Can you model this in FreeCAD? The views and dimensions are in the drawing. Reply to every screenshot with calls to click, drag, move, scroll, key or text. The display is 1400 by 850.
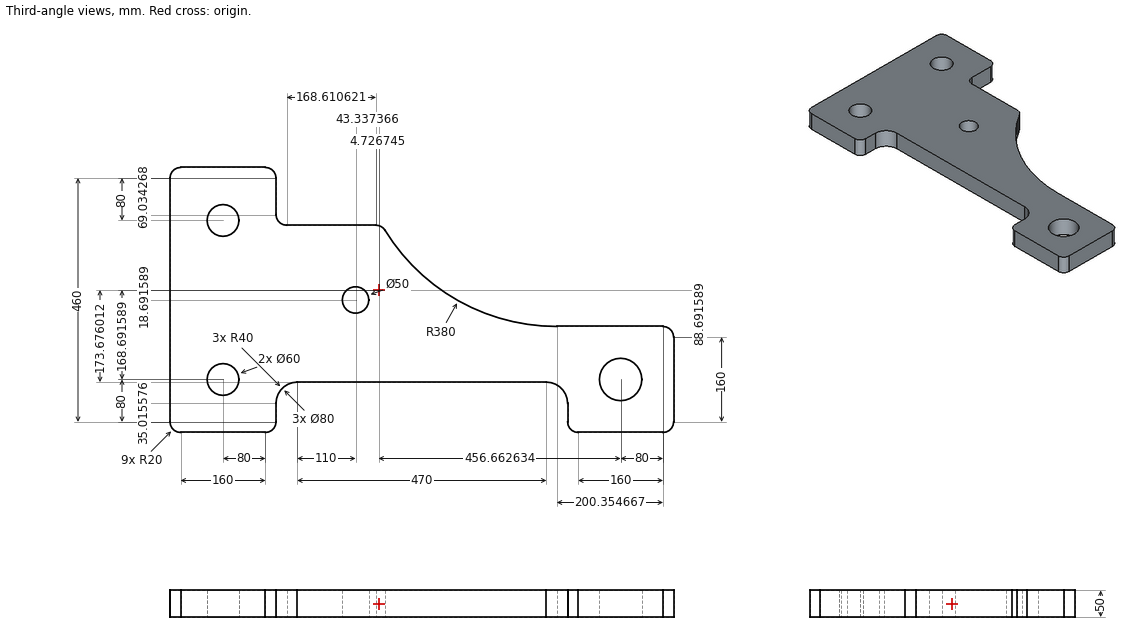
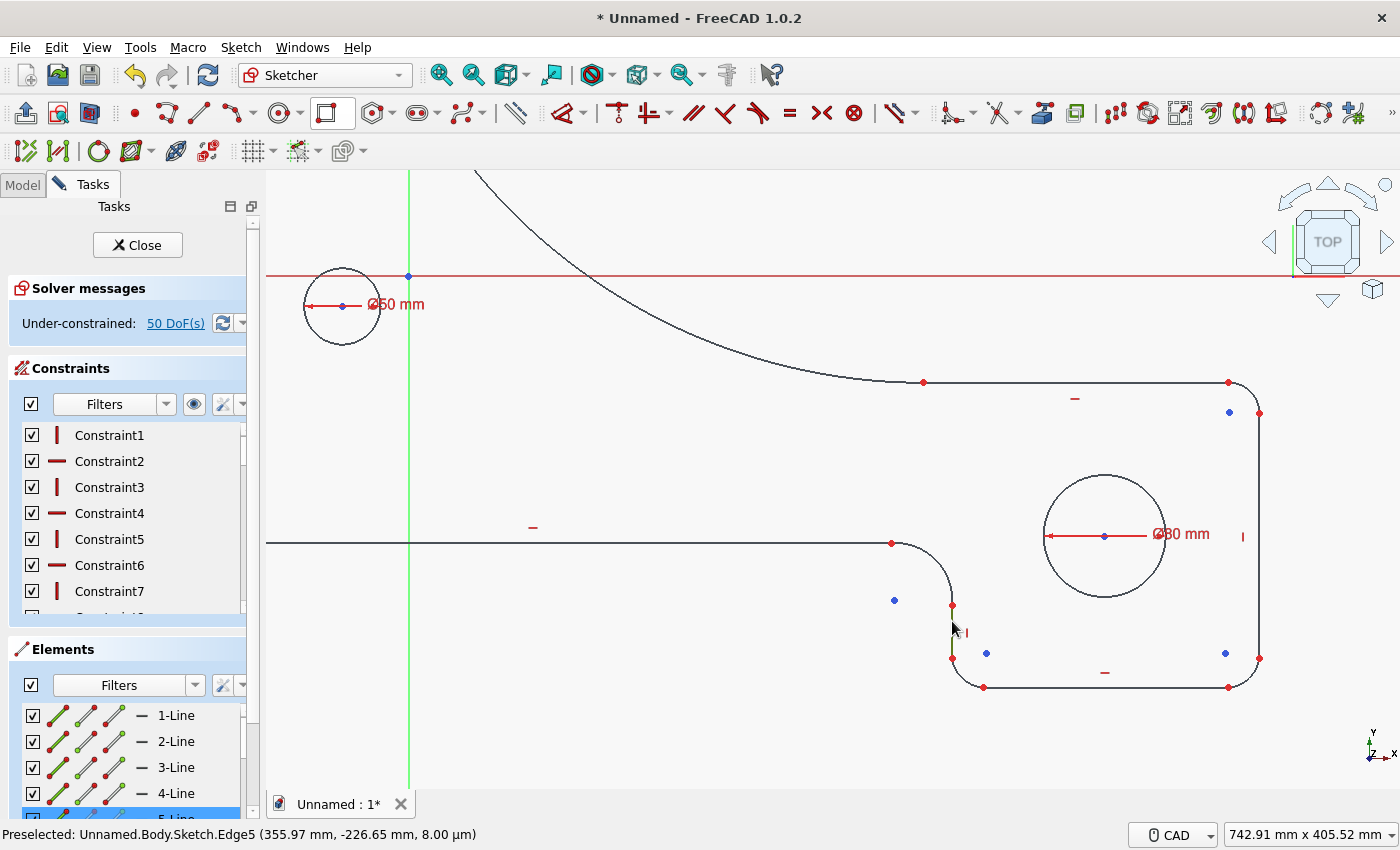
click(957, 672)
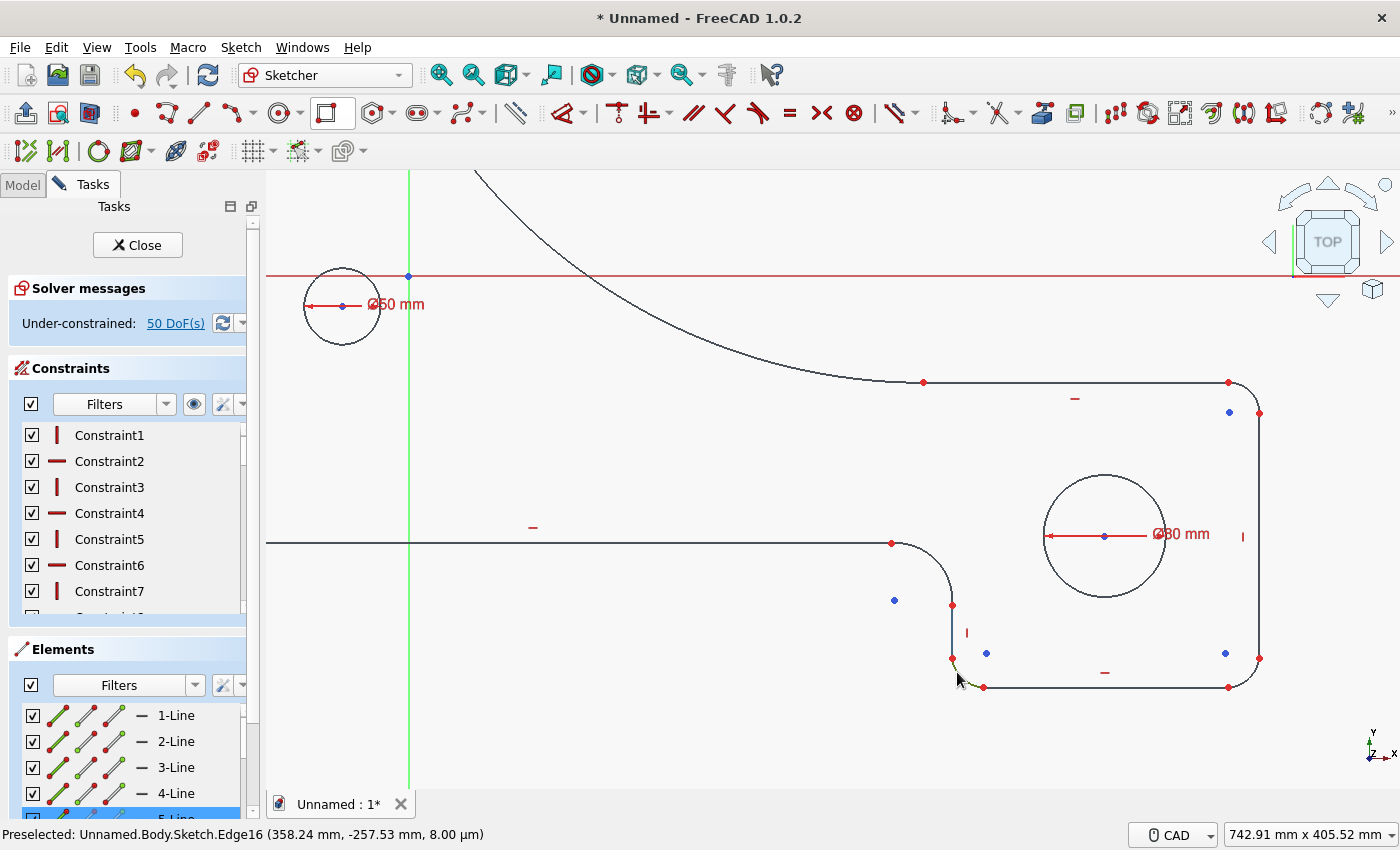
click(758, 114)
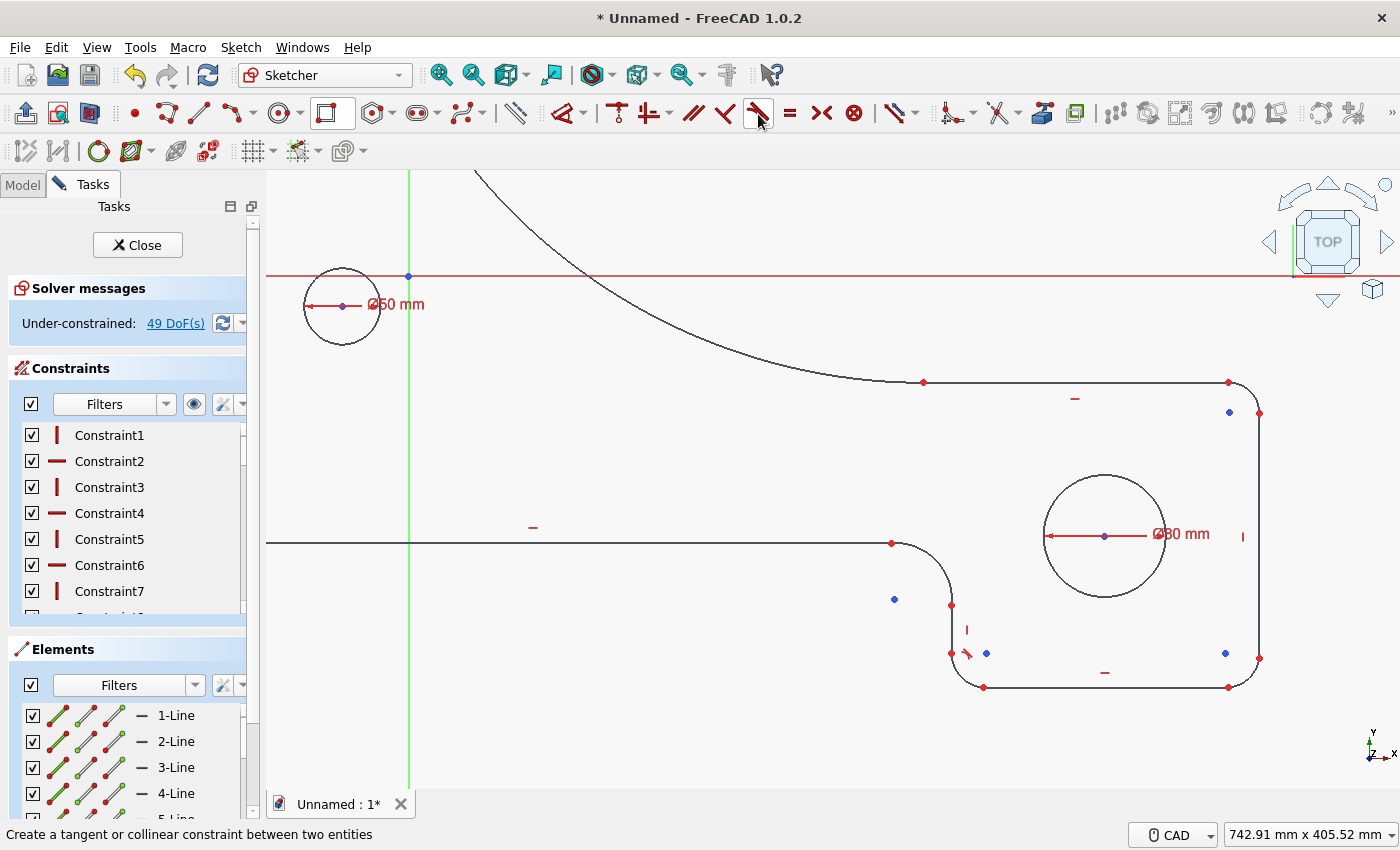
click(1057, 688)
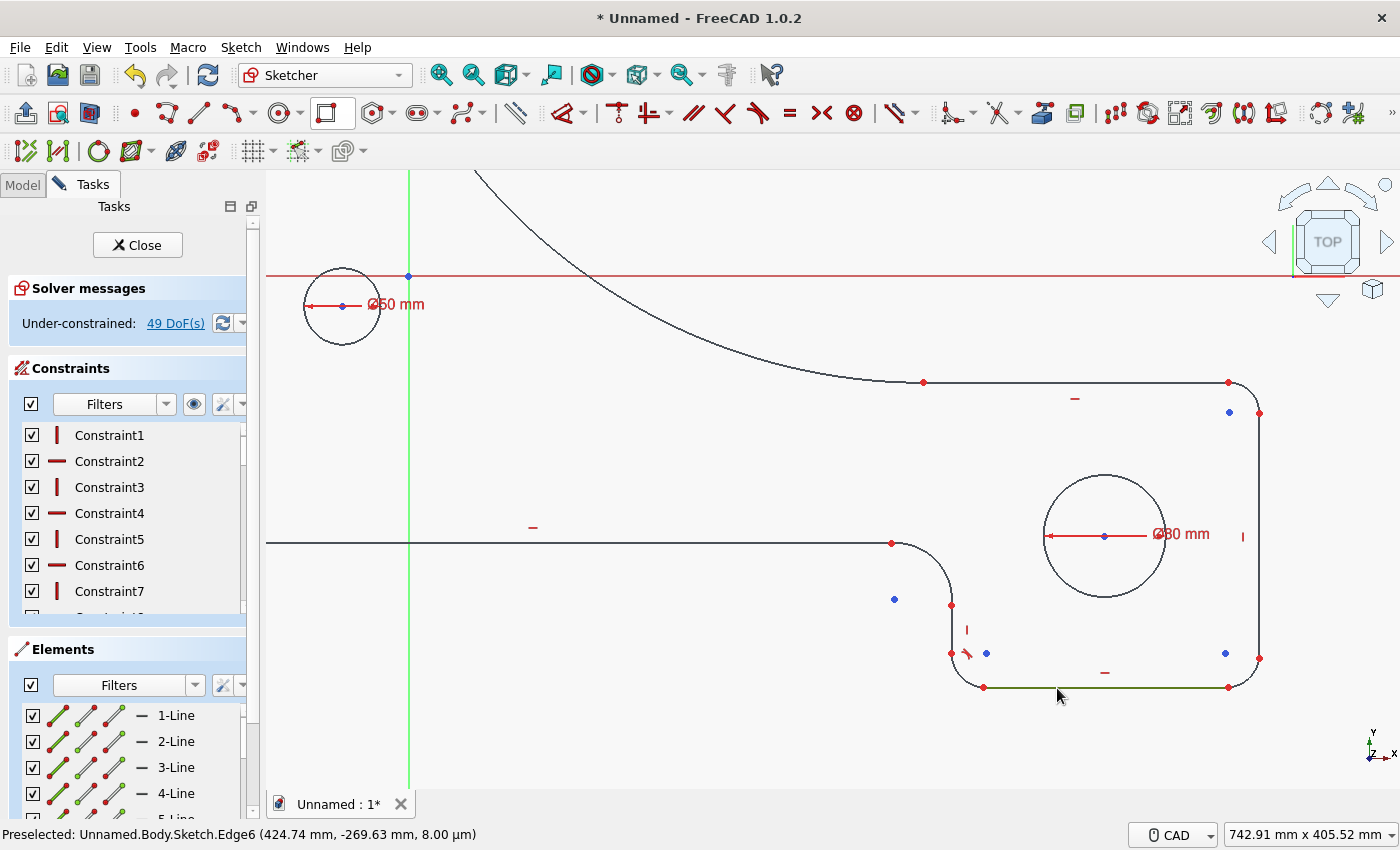
click(955, 668)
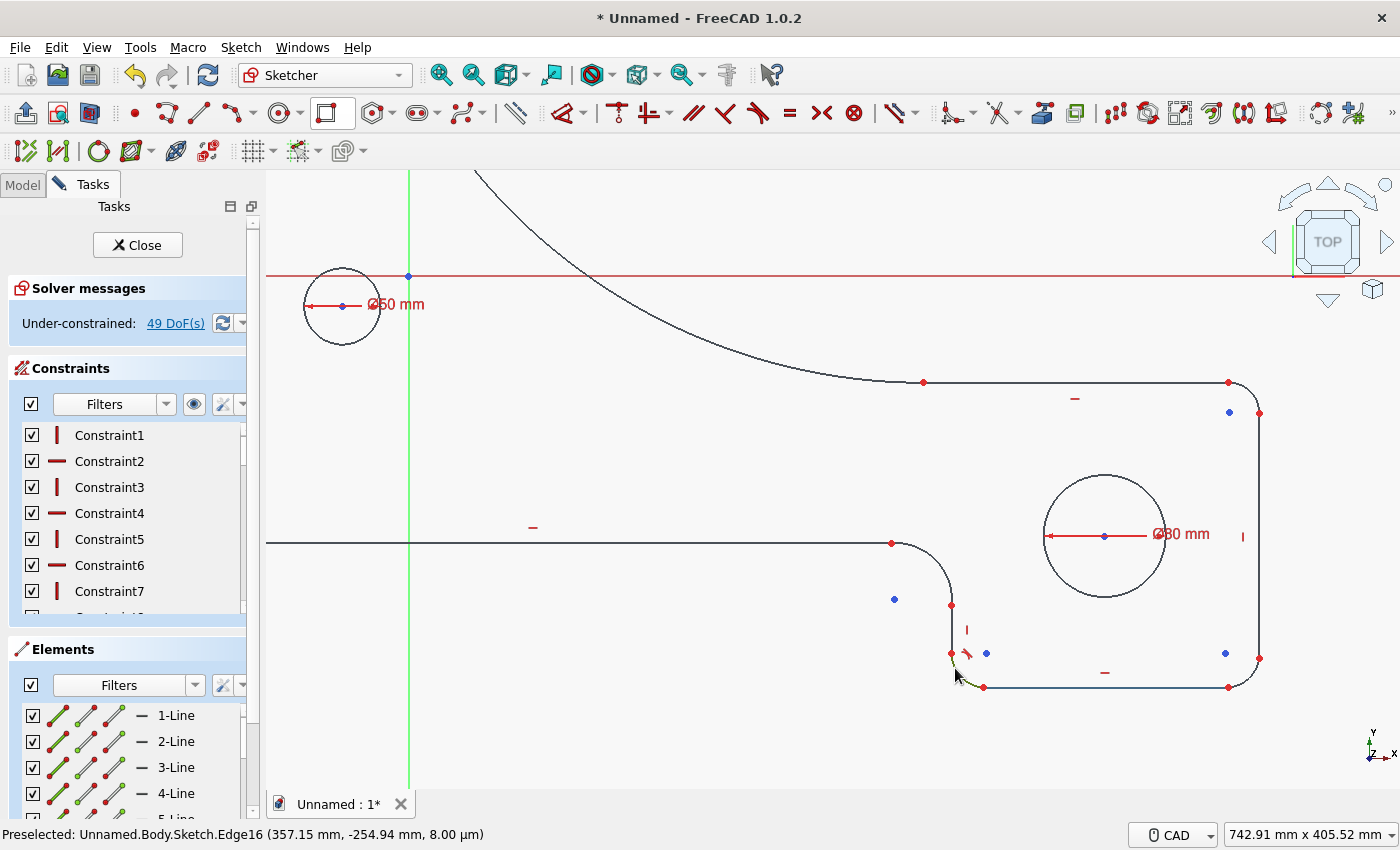
click(758, 114)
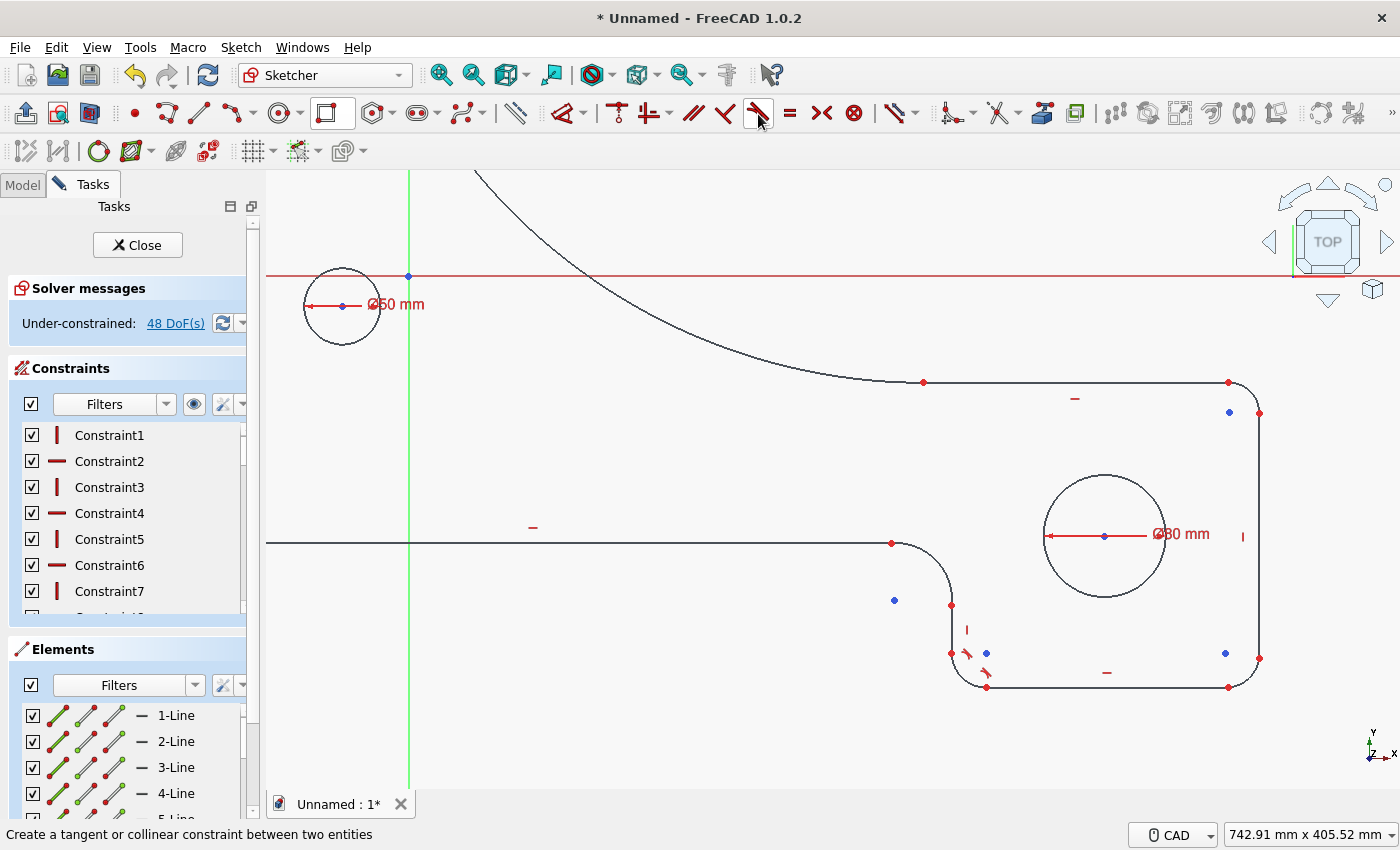
click(1059, 688)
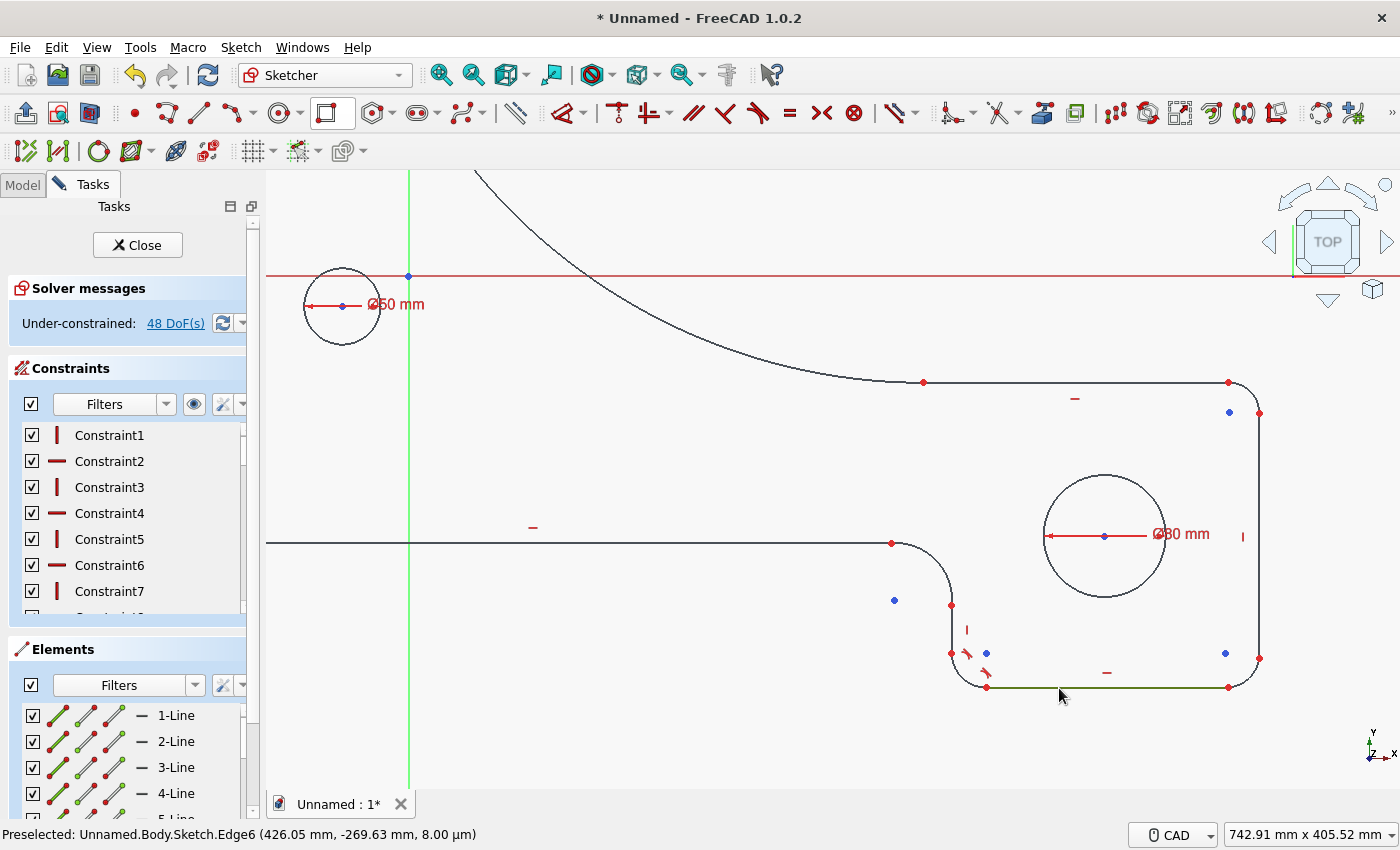
scroll(953, 622, down, 4)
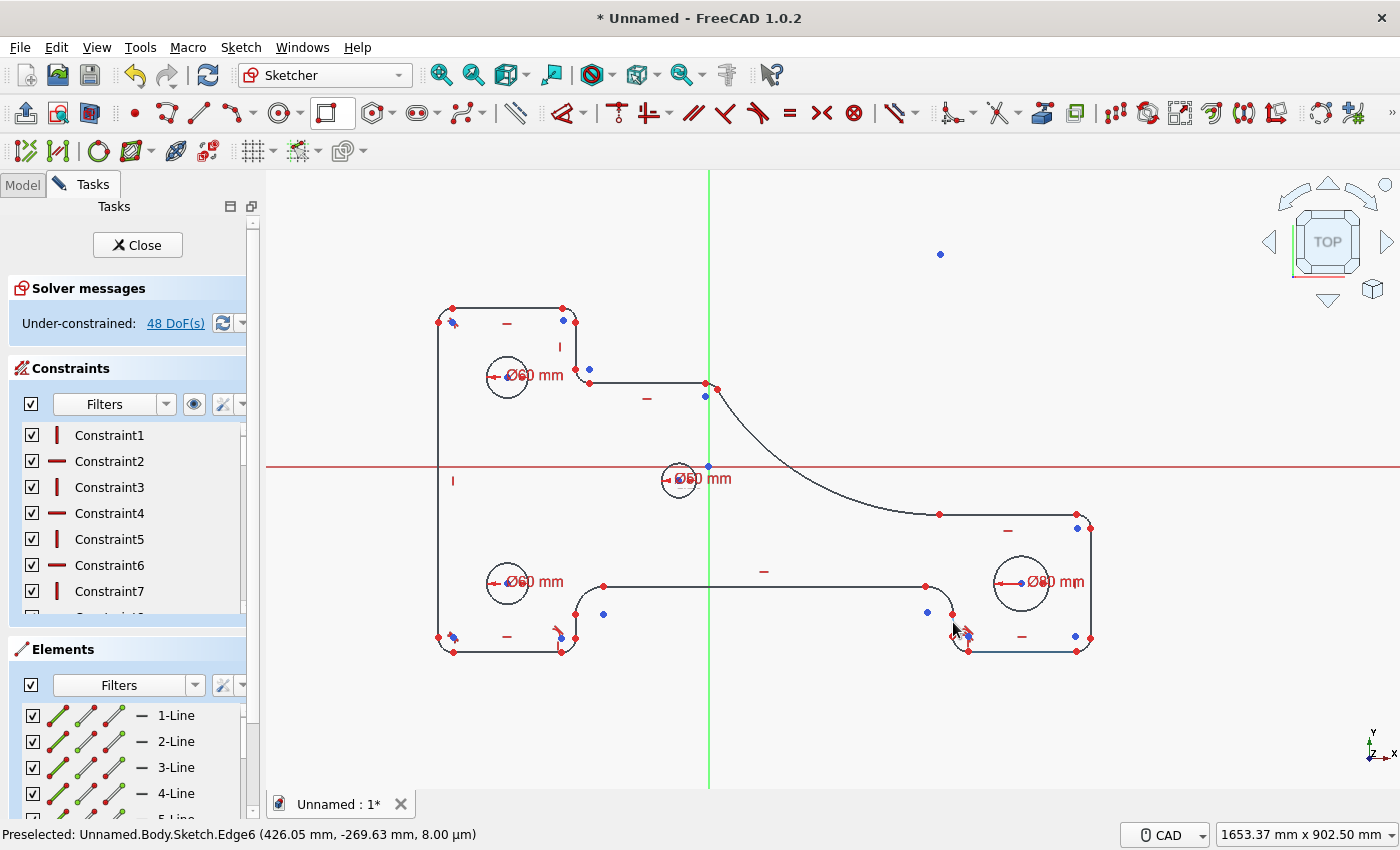
scroll(1083, 650, up, 5)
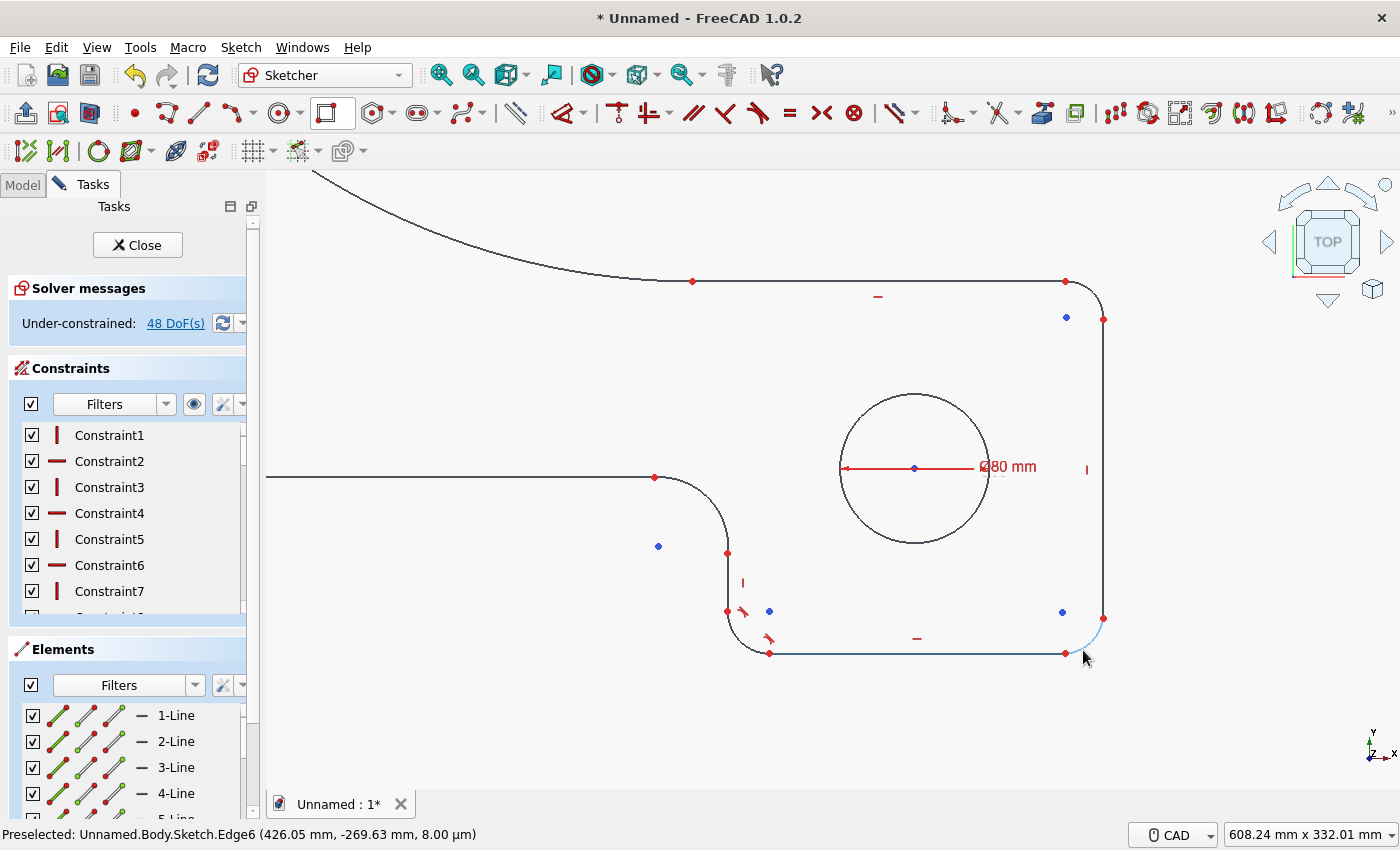
click(1081, 649)